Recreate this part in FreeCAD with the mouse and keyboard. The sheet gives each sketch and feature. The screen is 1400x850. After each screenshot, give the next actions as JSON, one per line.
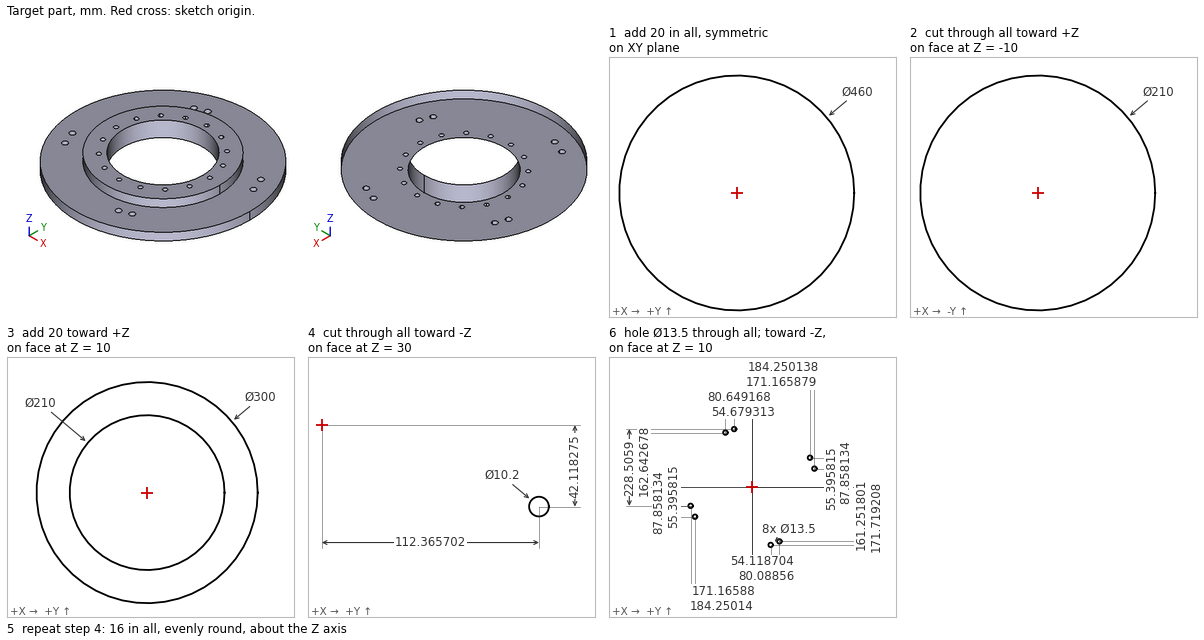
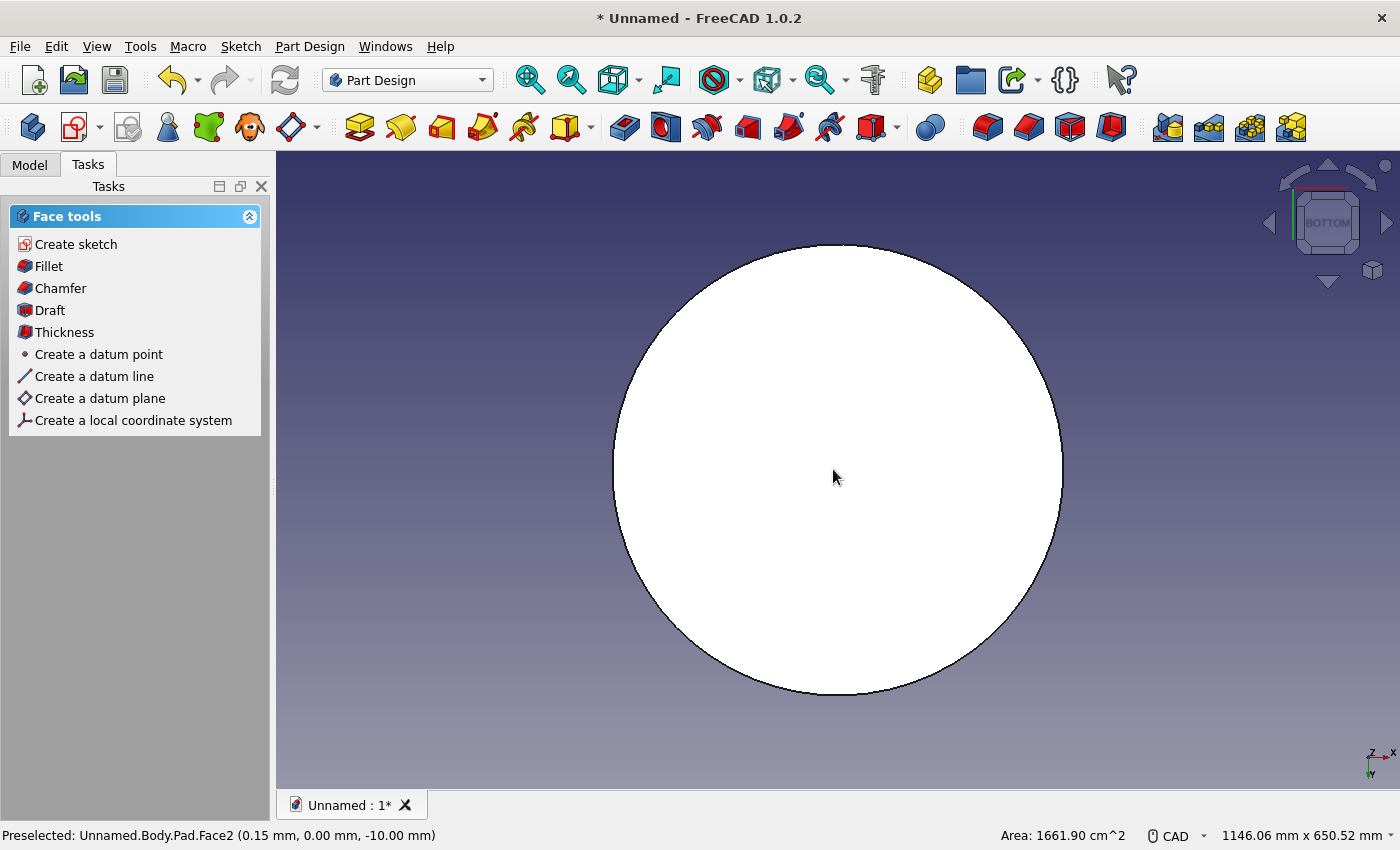
{"action": "left_click", "coordinate": [74, 128]}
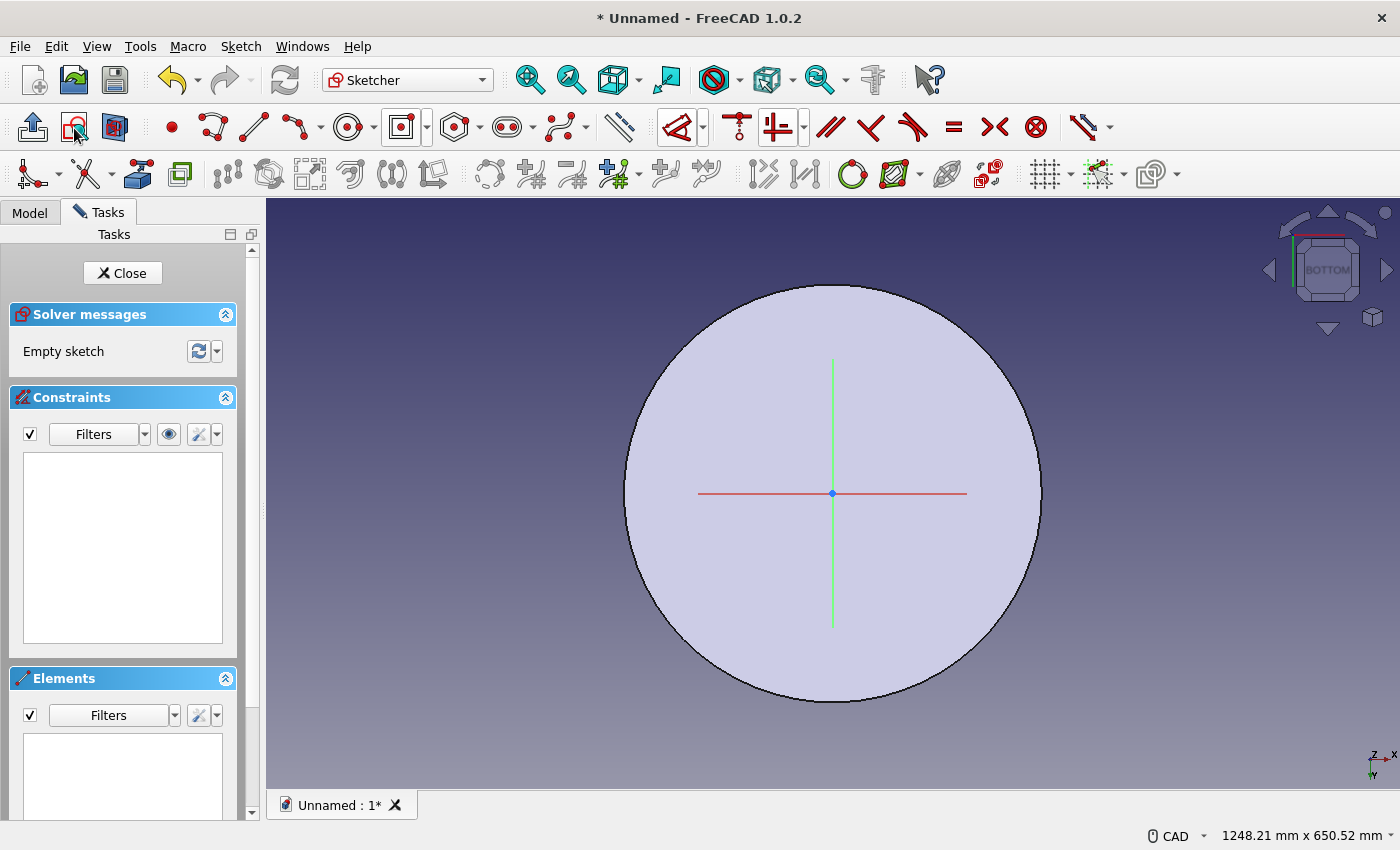
{"action": "scroll", "coordinate": [916, 494], "scroll_direction": "up", "scroll_amount": 3}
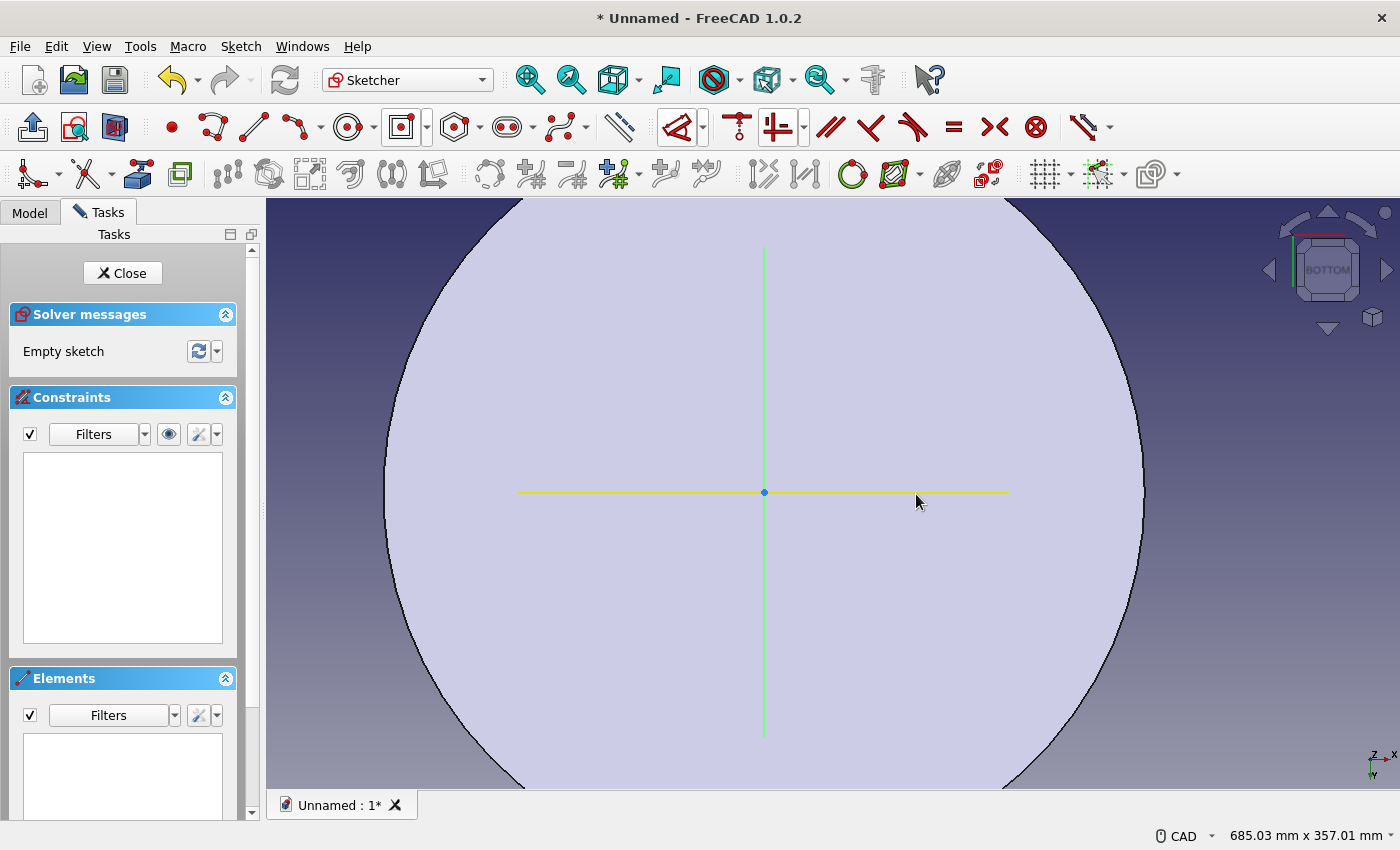
{"action": "key", "text": "g c"}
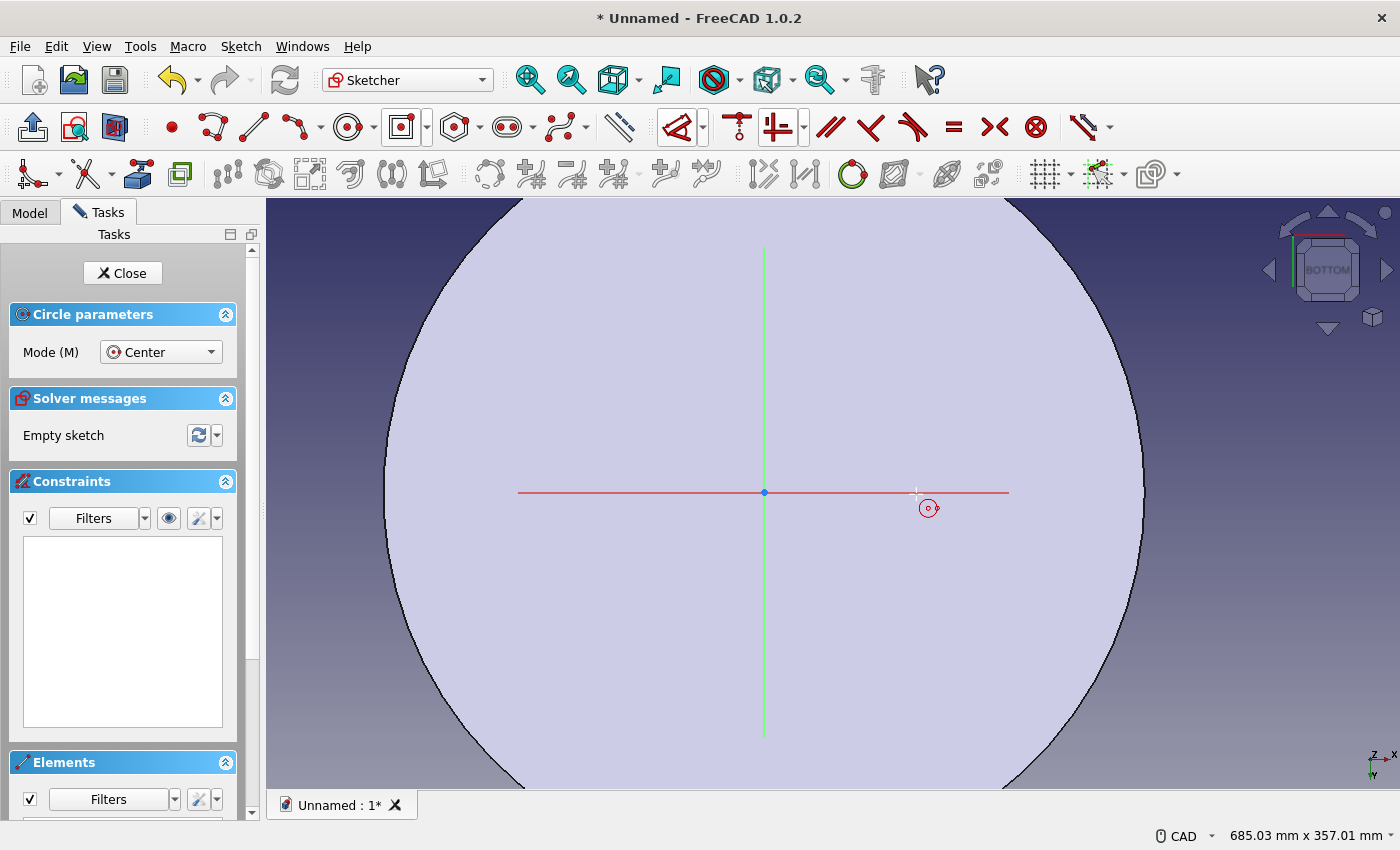
{"action": "left_click", "coordinate": [764, 493]}
{"action": "mouse_move", "coordinate": [887, 370]}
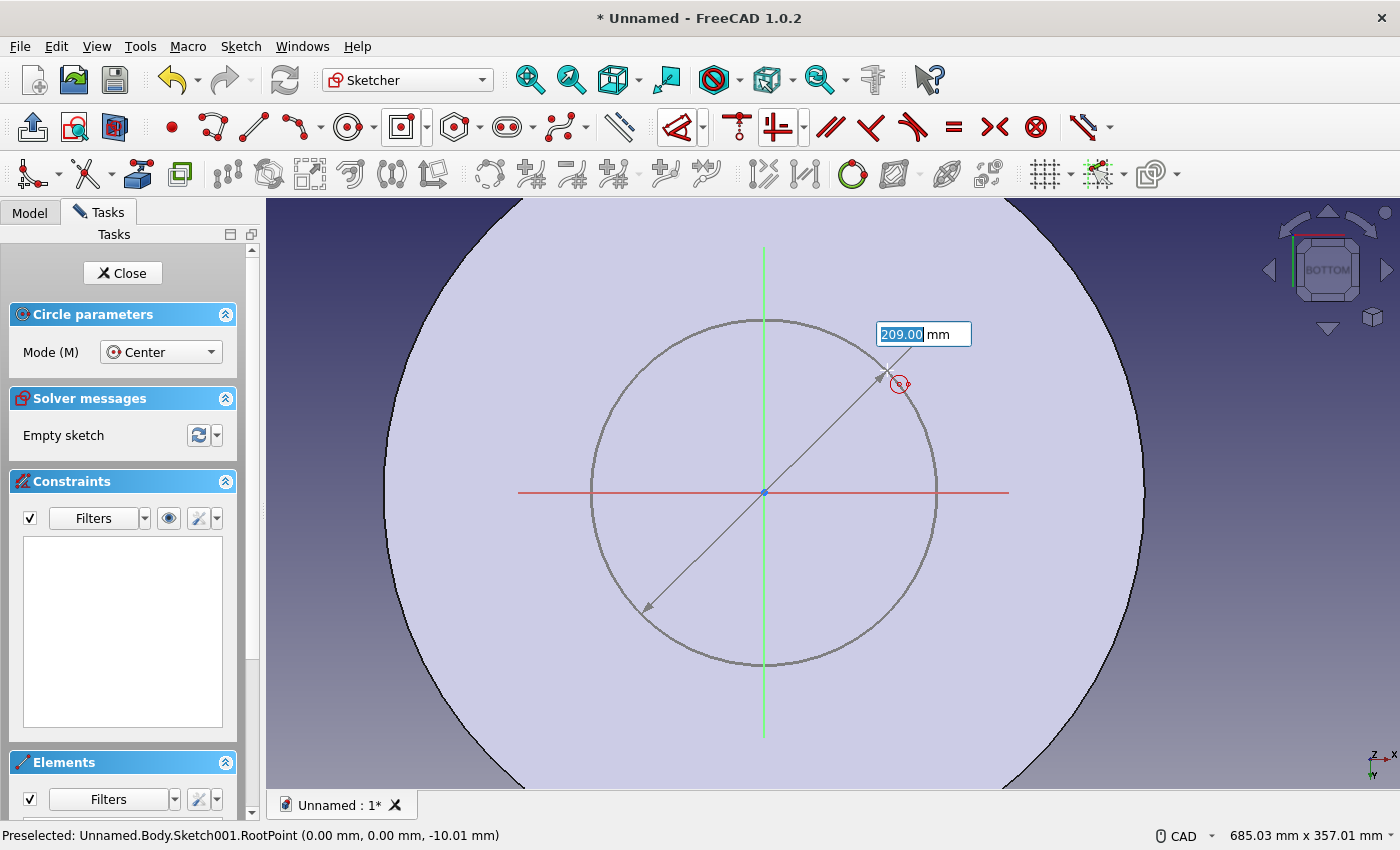
{"action": "type", "text": "210"}
{"action": "key", "text": "Return"}
{"action": "key", "text": "Escape"}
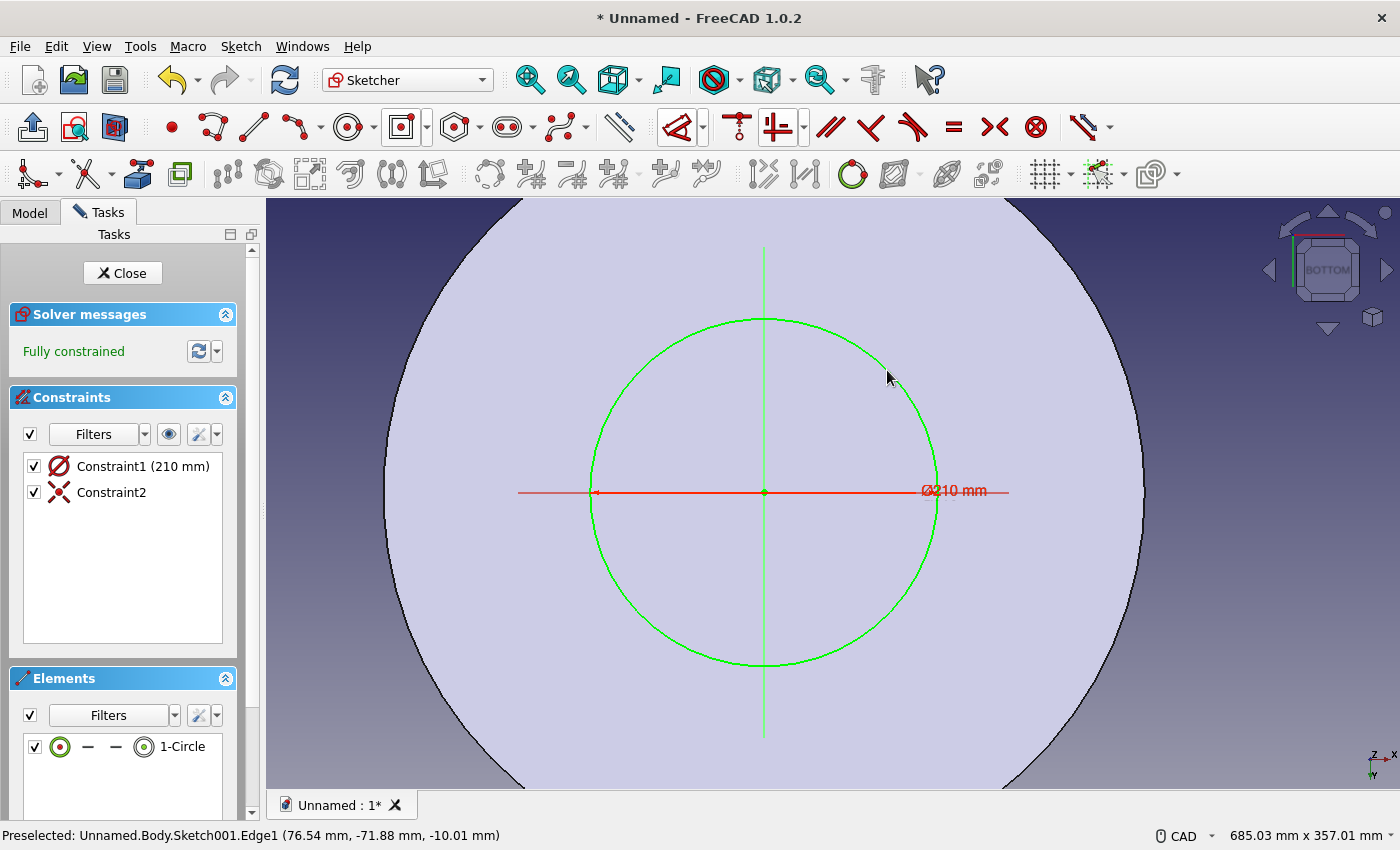
{"action": "left_click", "coordinate": [123, 273]}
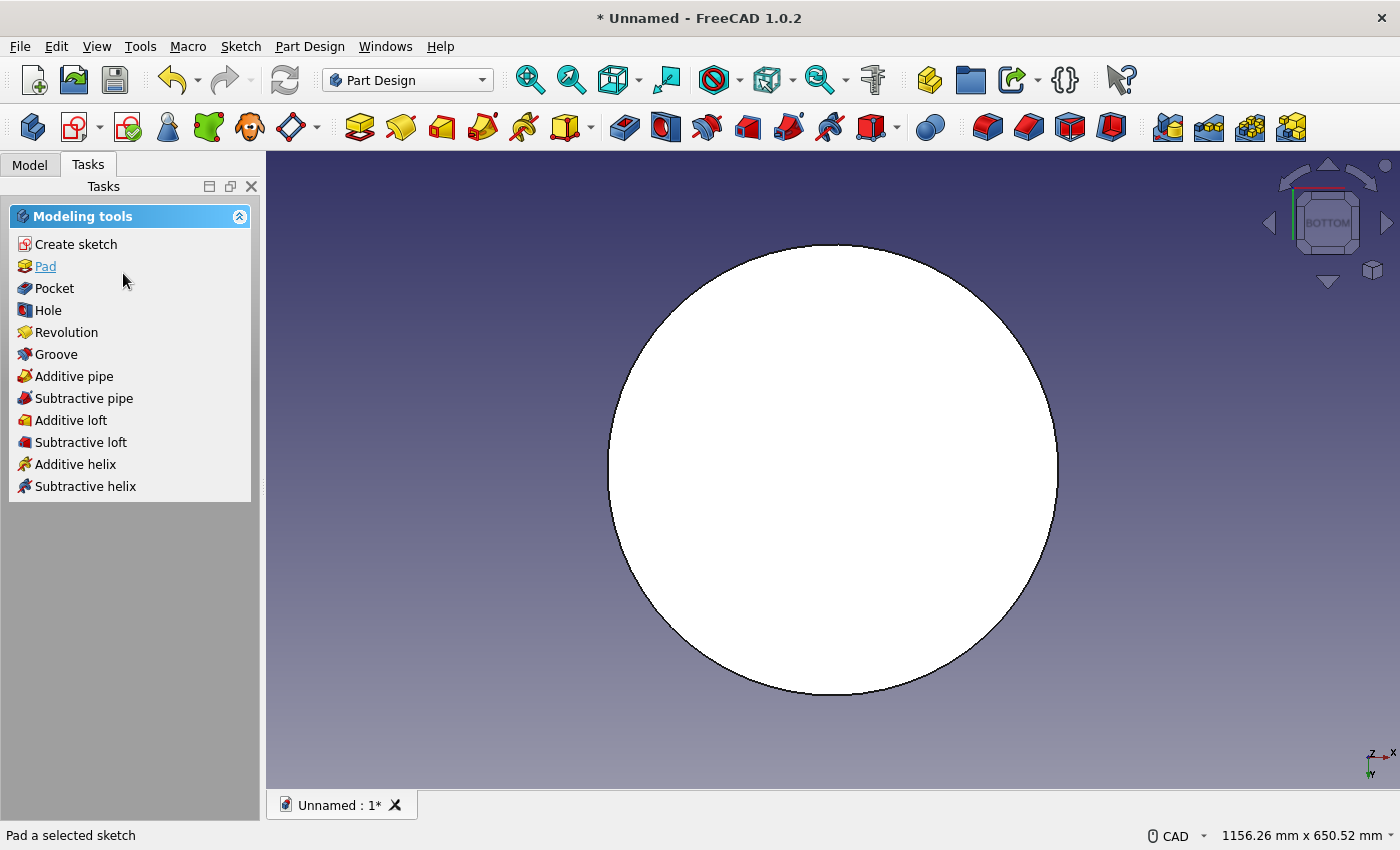
{"action": "left_click", "coordinate": [625, 128]}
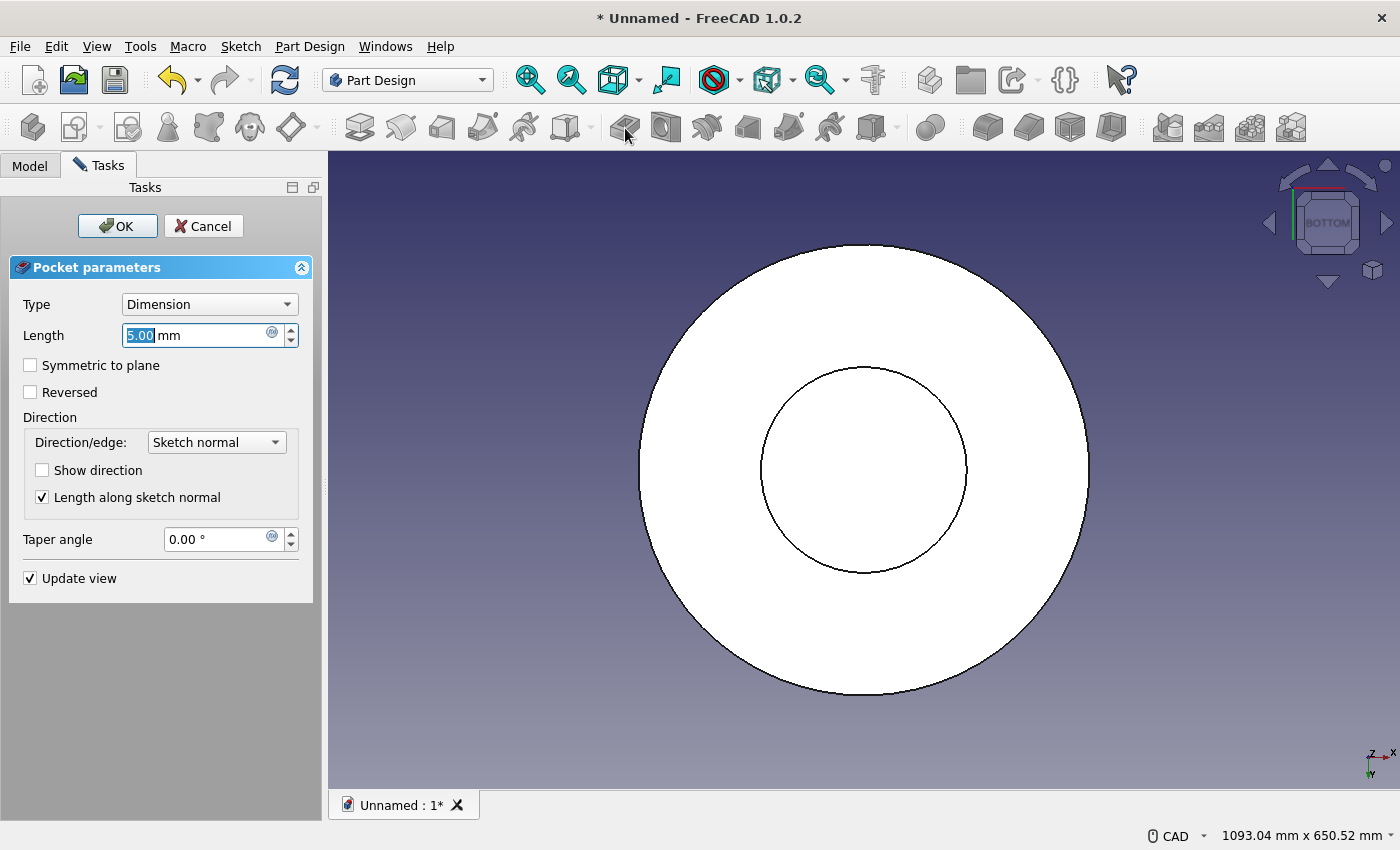
{"action": "left_click", "coordinate": [210, 304]}